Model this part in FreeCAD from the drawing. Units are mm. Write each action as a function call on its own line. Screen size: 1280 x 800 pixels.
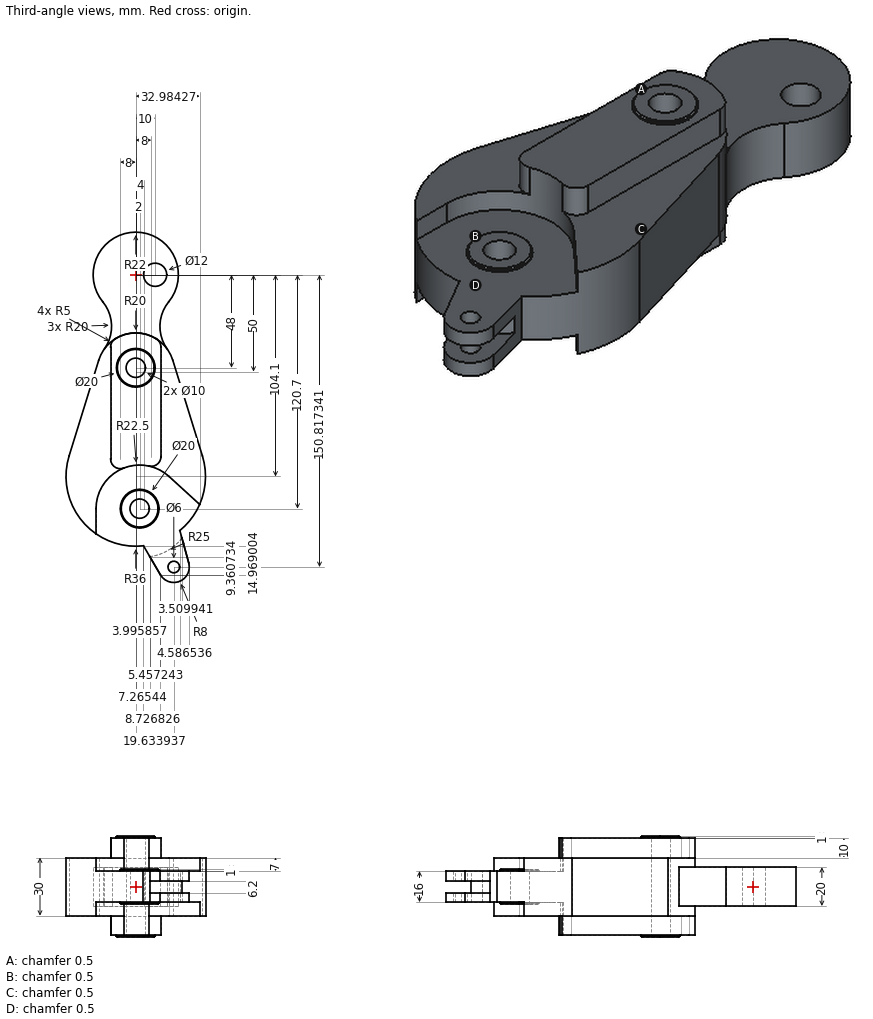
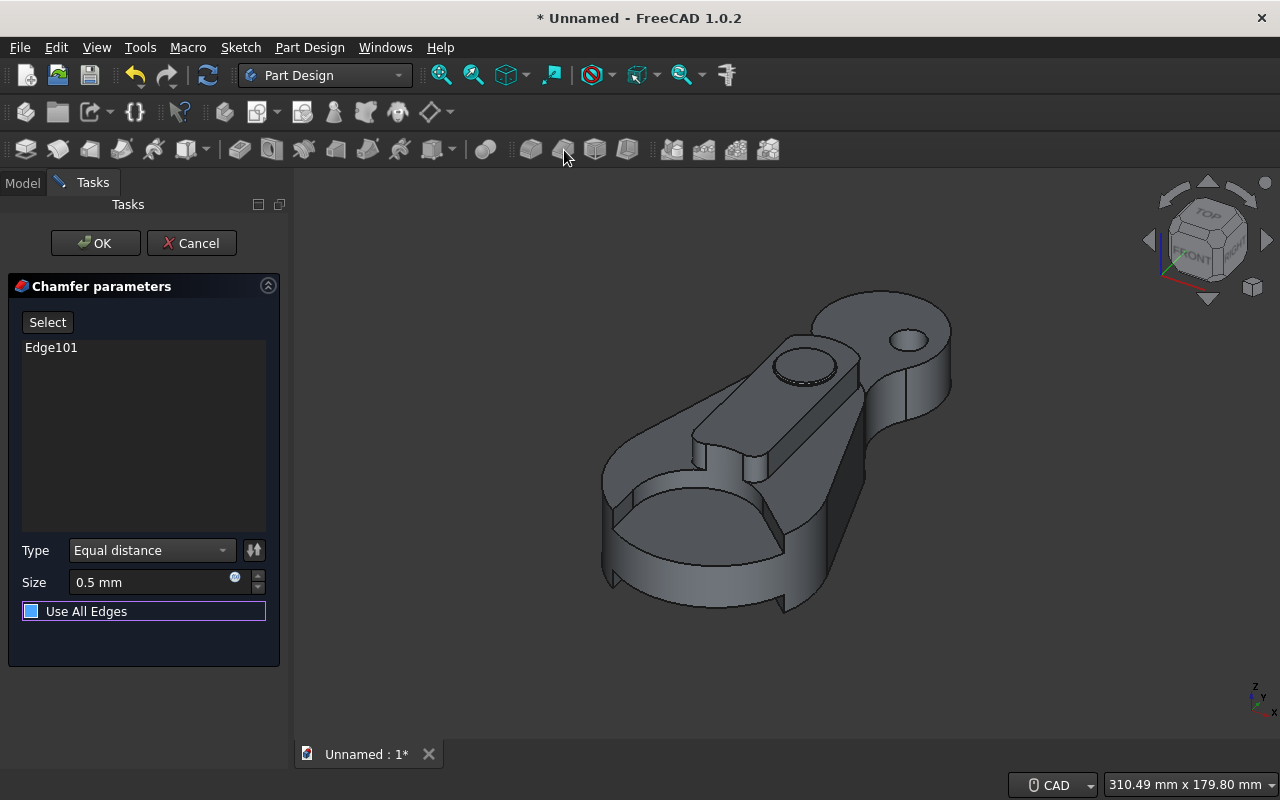
click(96, 243)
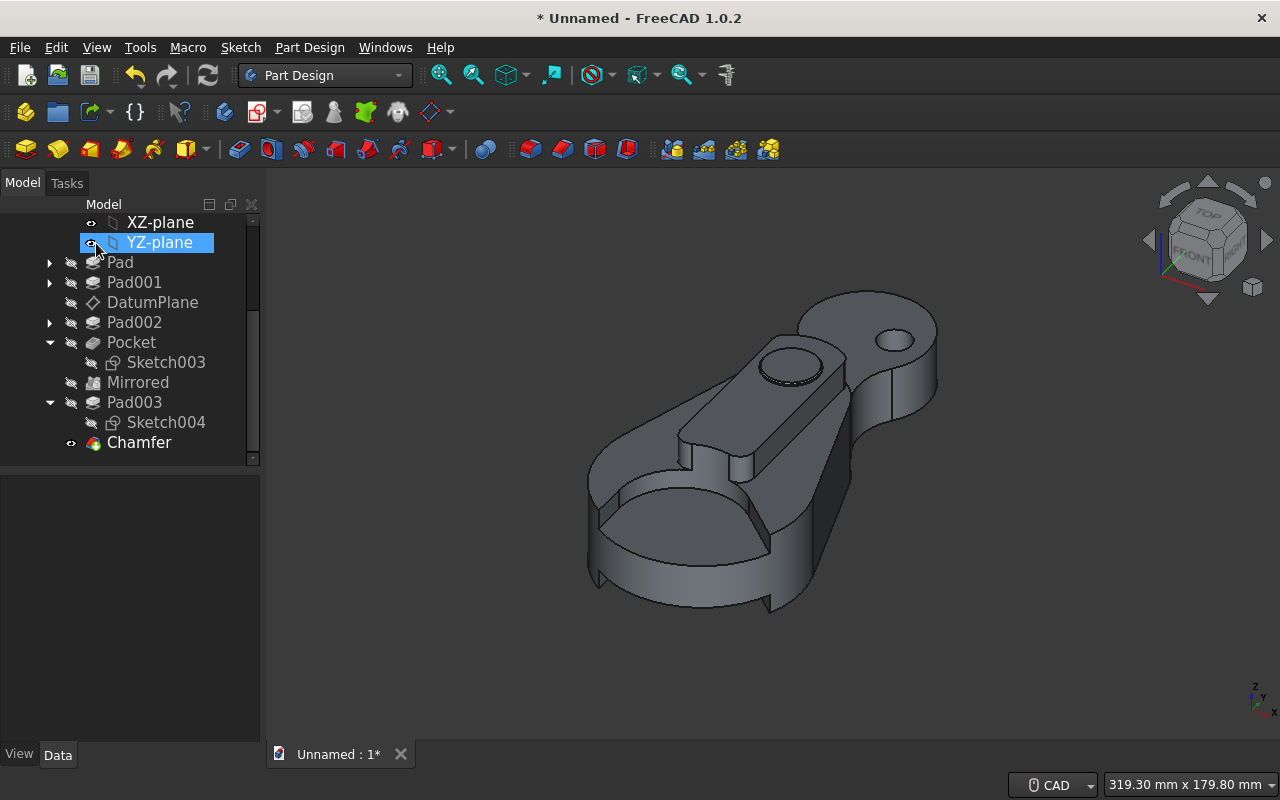
click(674, 522)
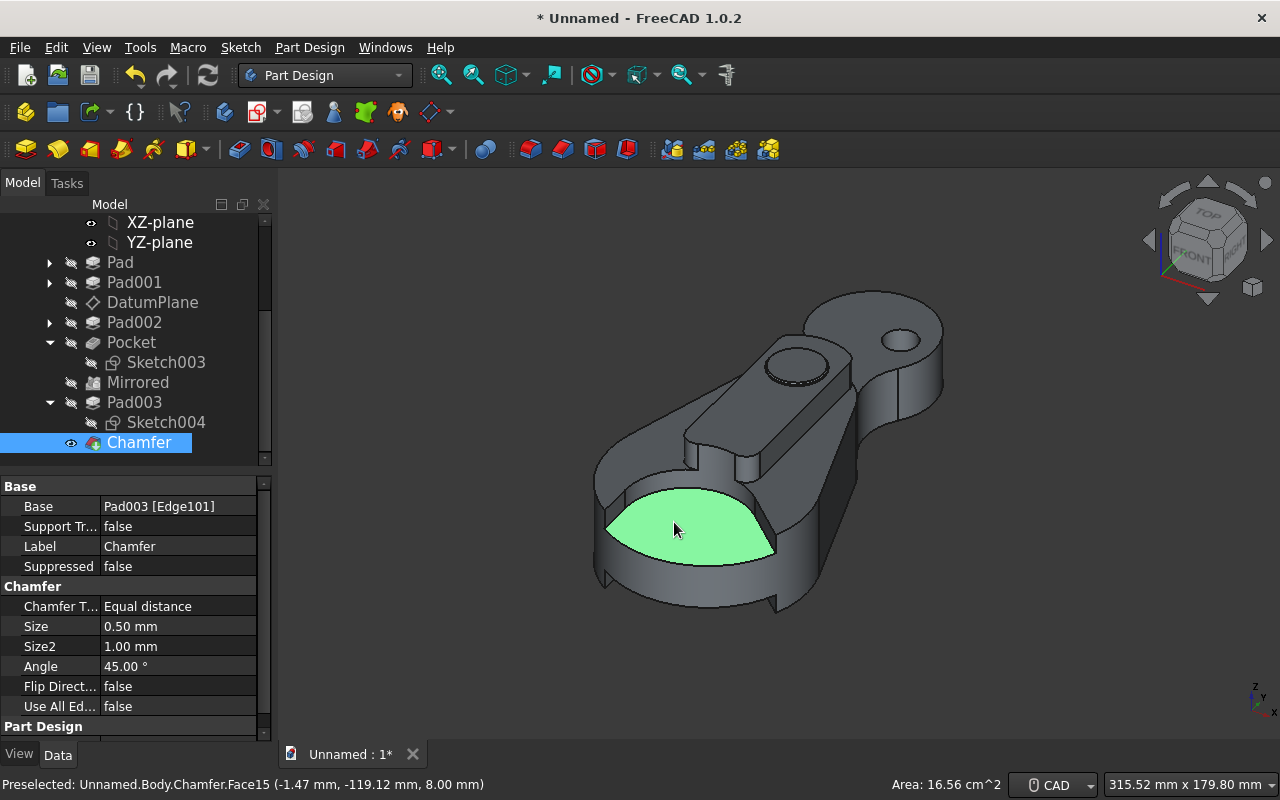
click(258, 112)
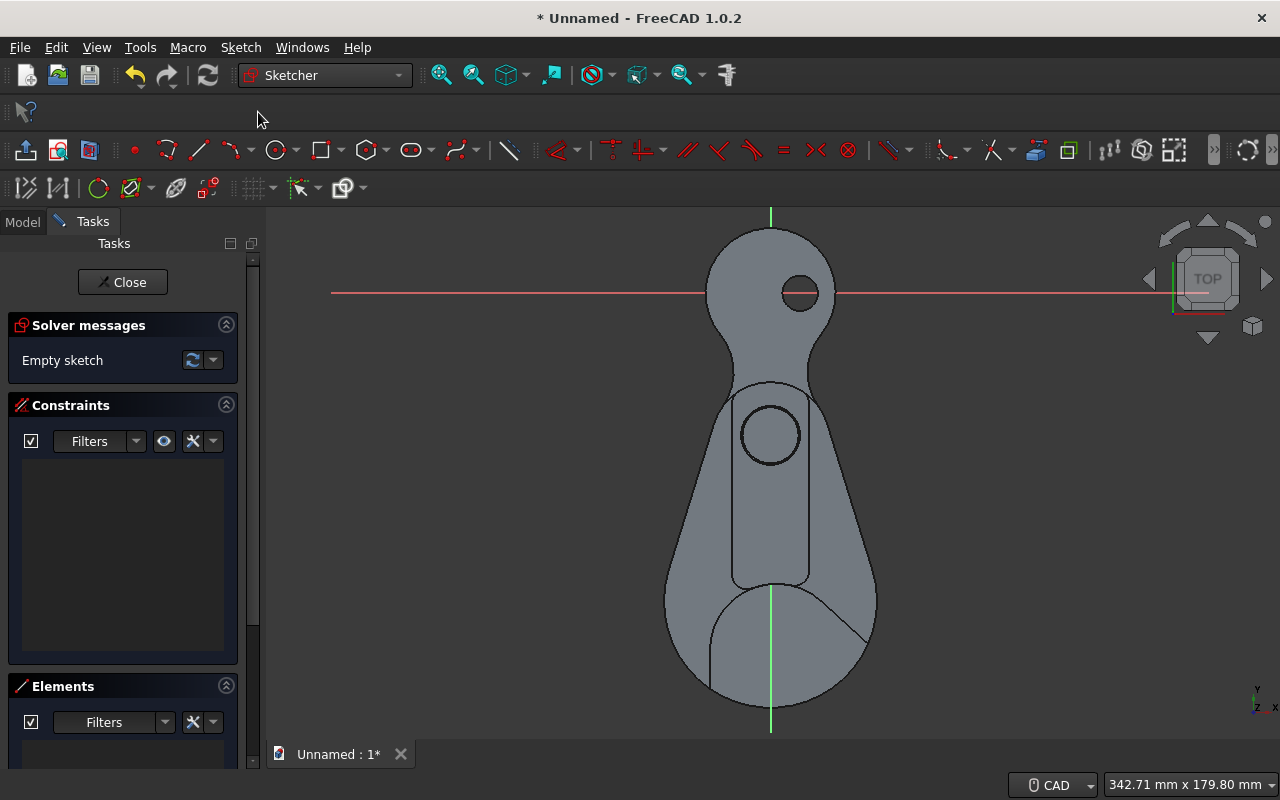
click(90, 150)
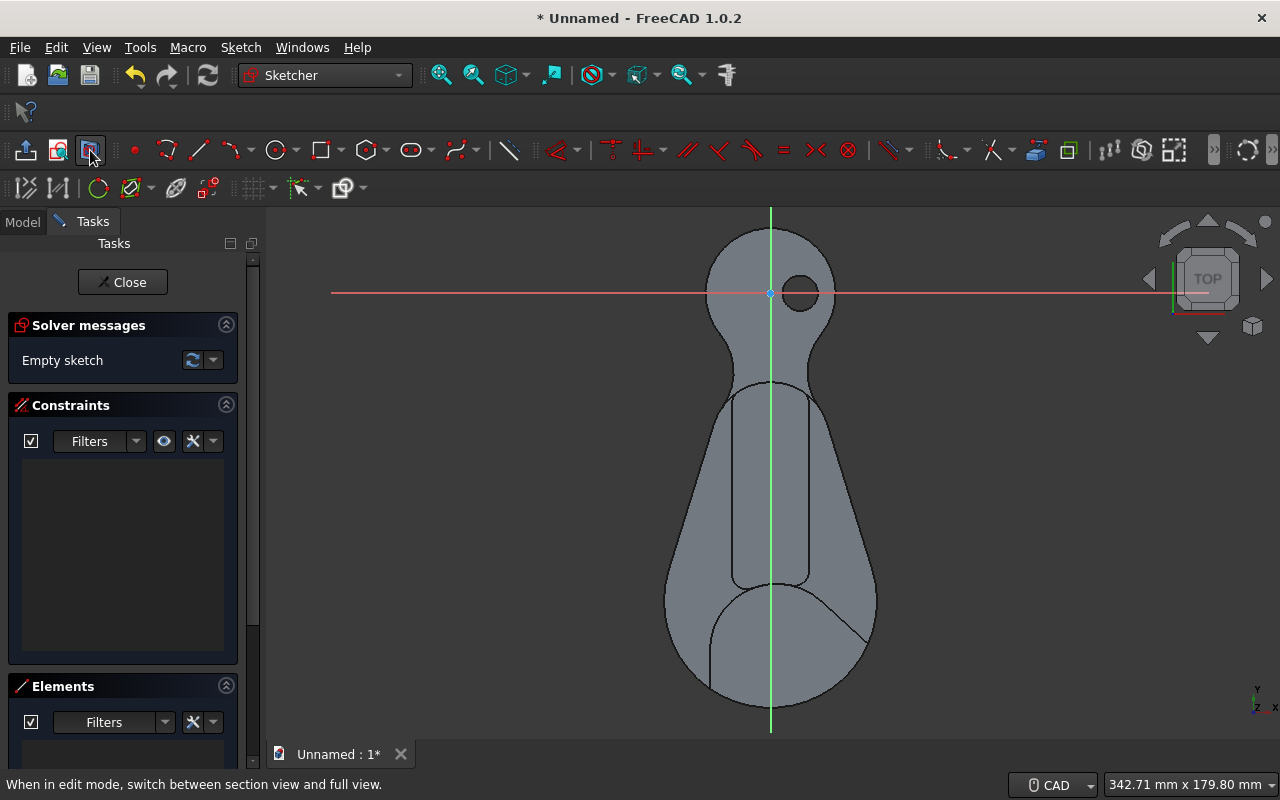
scroll(791, 686, up, 9)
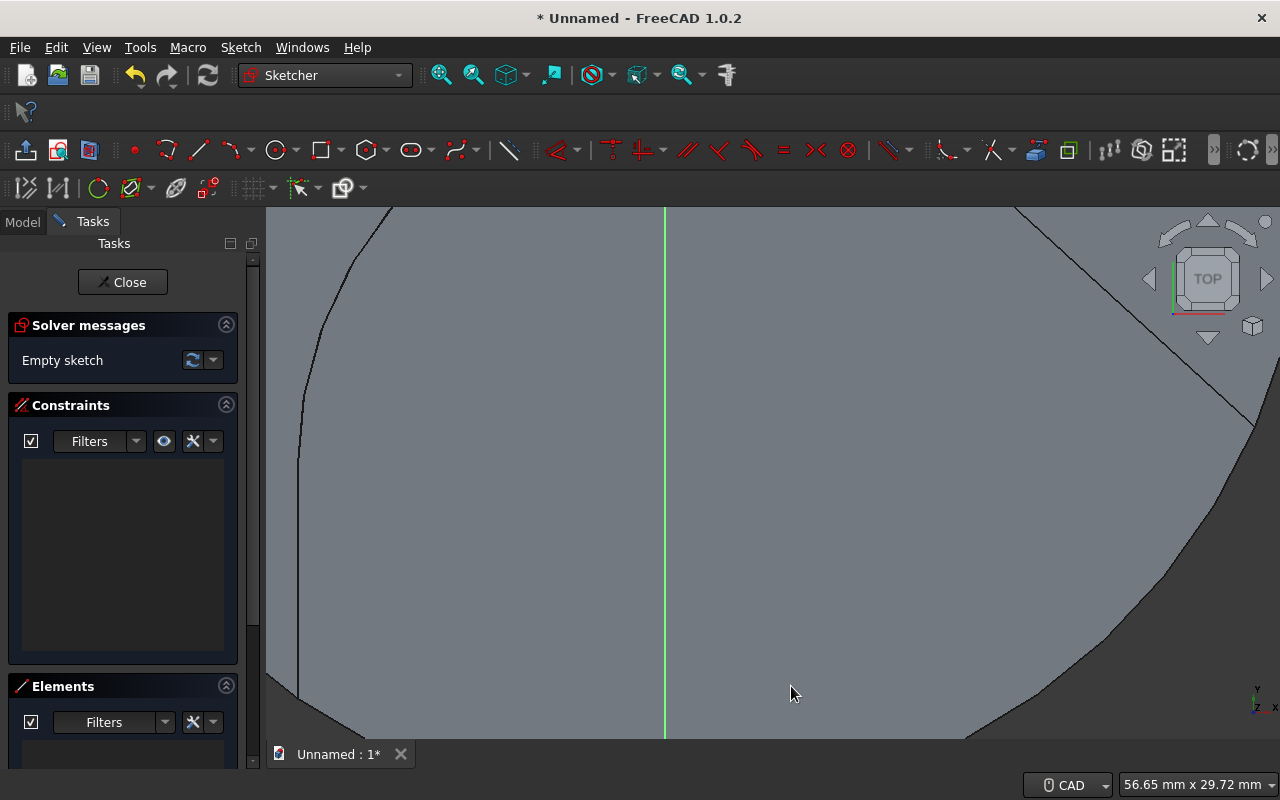
click(276, 150)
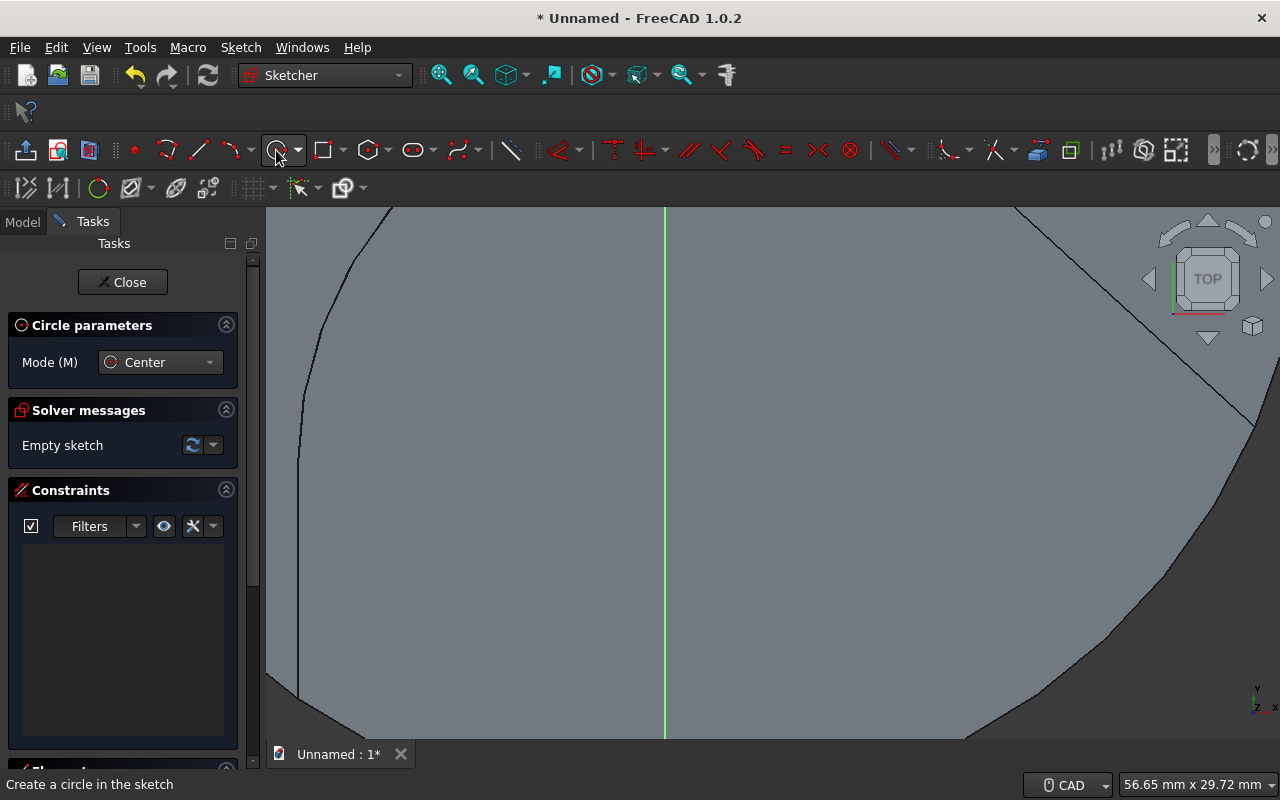
click(701, 466)
click(827, 340)
key(Escape)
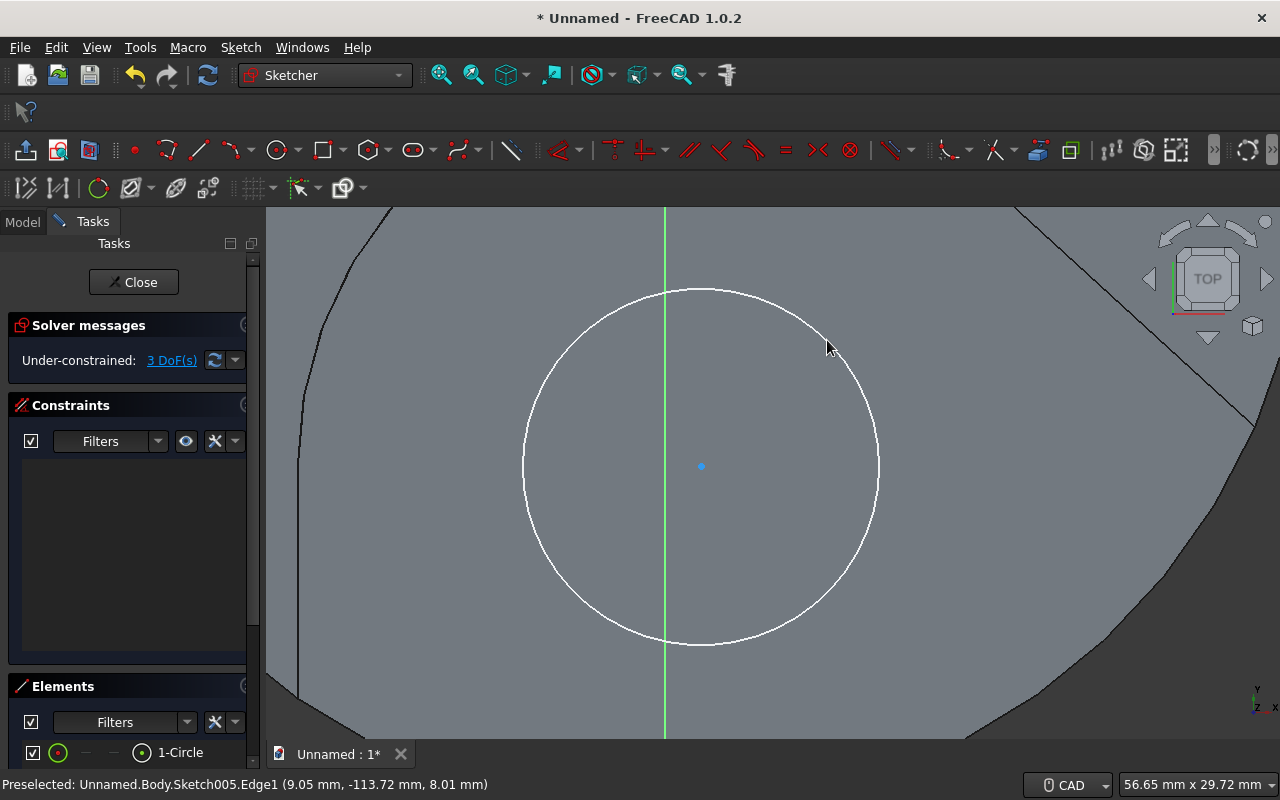
click(558, 150)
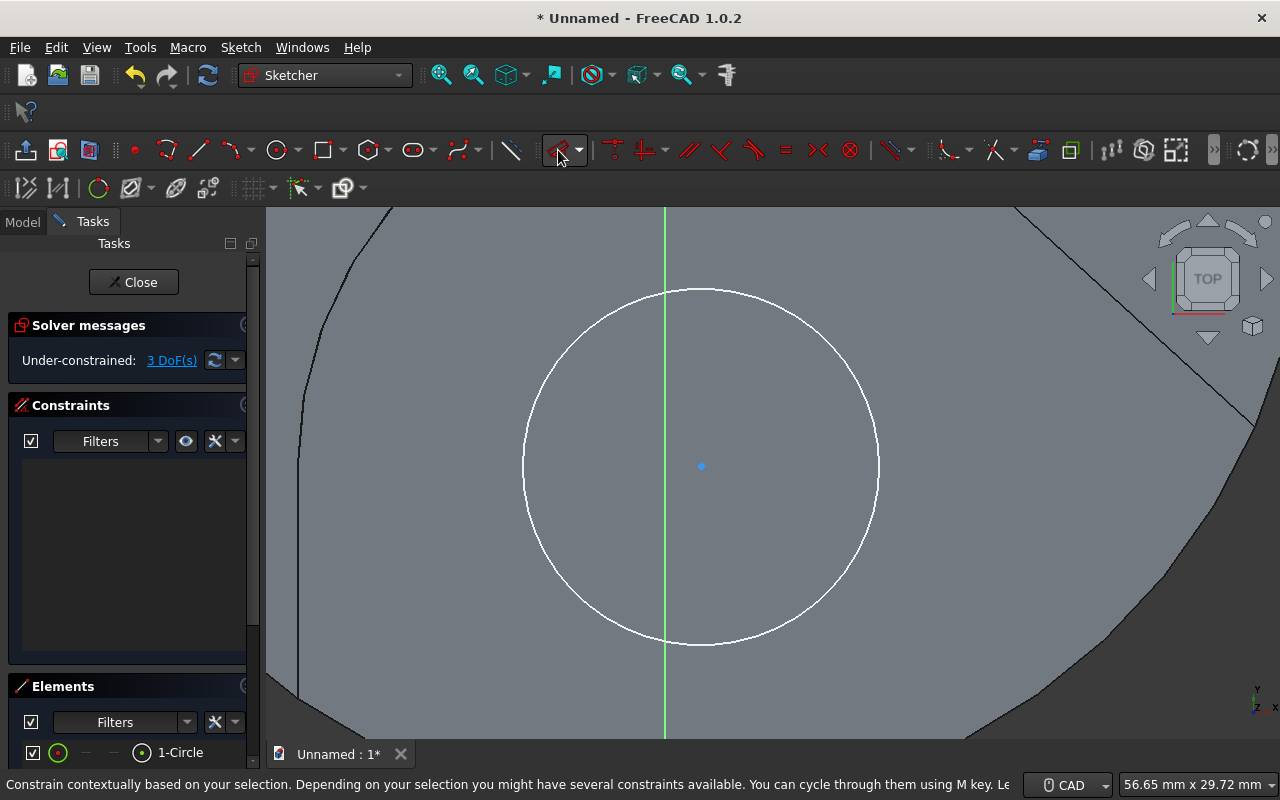
click(827, 341)
click(850, 318)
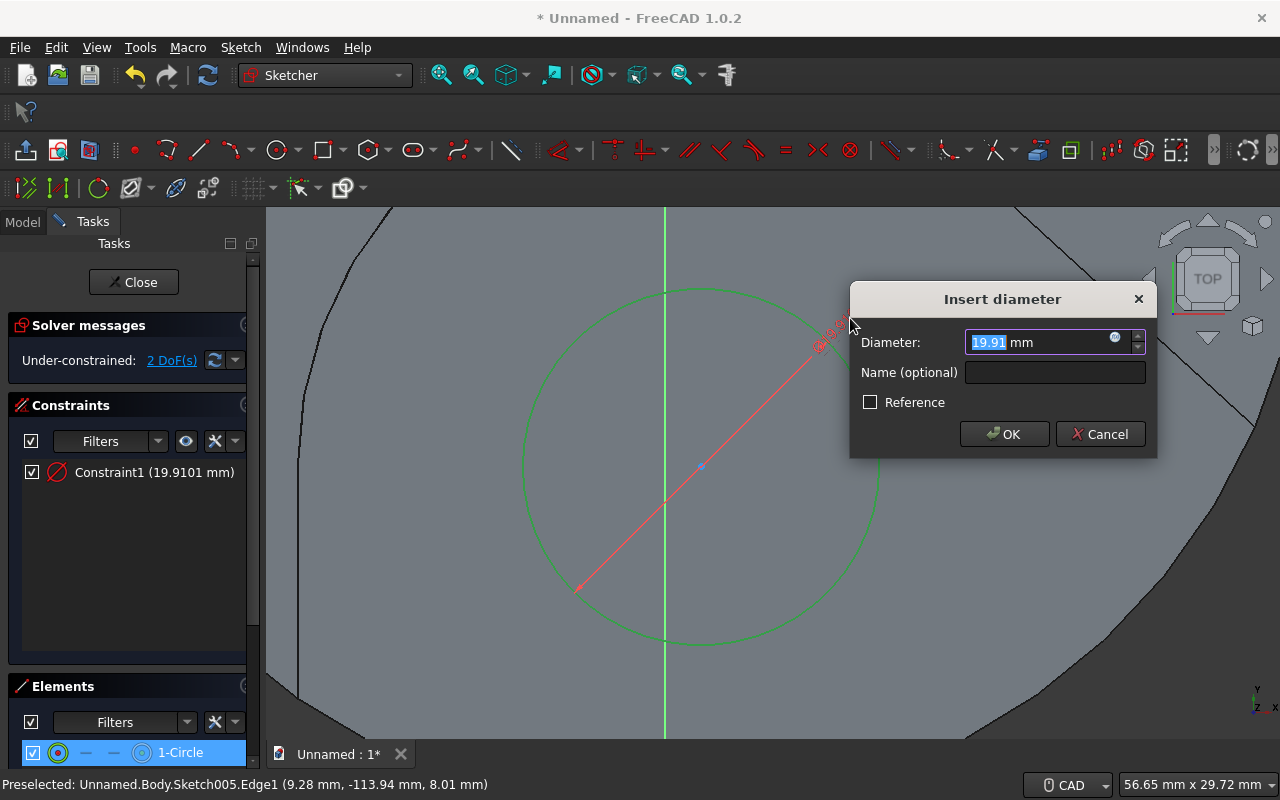
text(20)
key(Return)